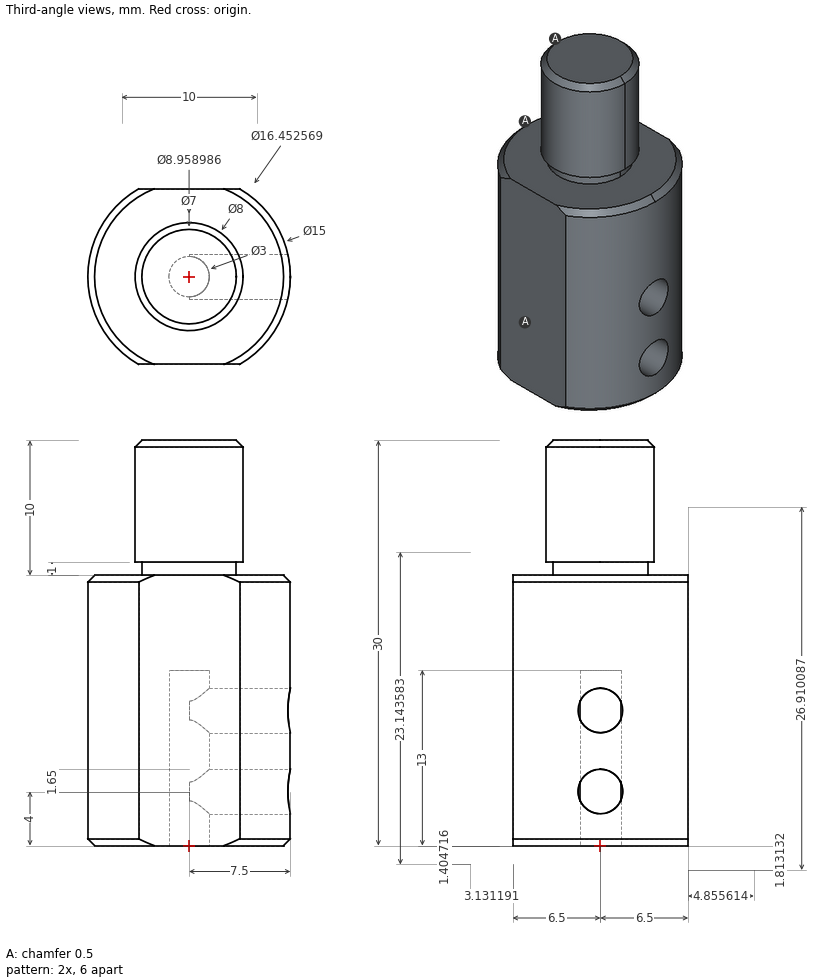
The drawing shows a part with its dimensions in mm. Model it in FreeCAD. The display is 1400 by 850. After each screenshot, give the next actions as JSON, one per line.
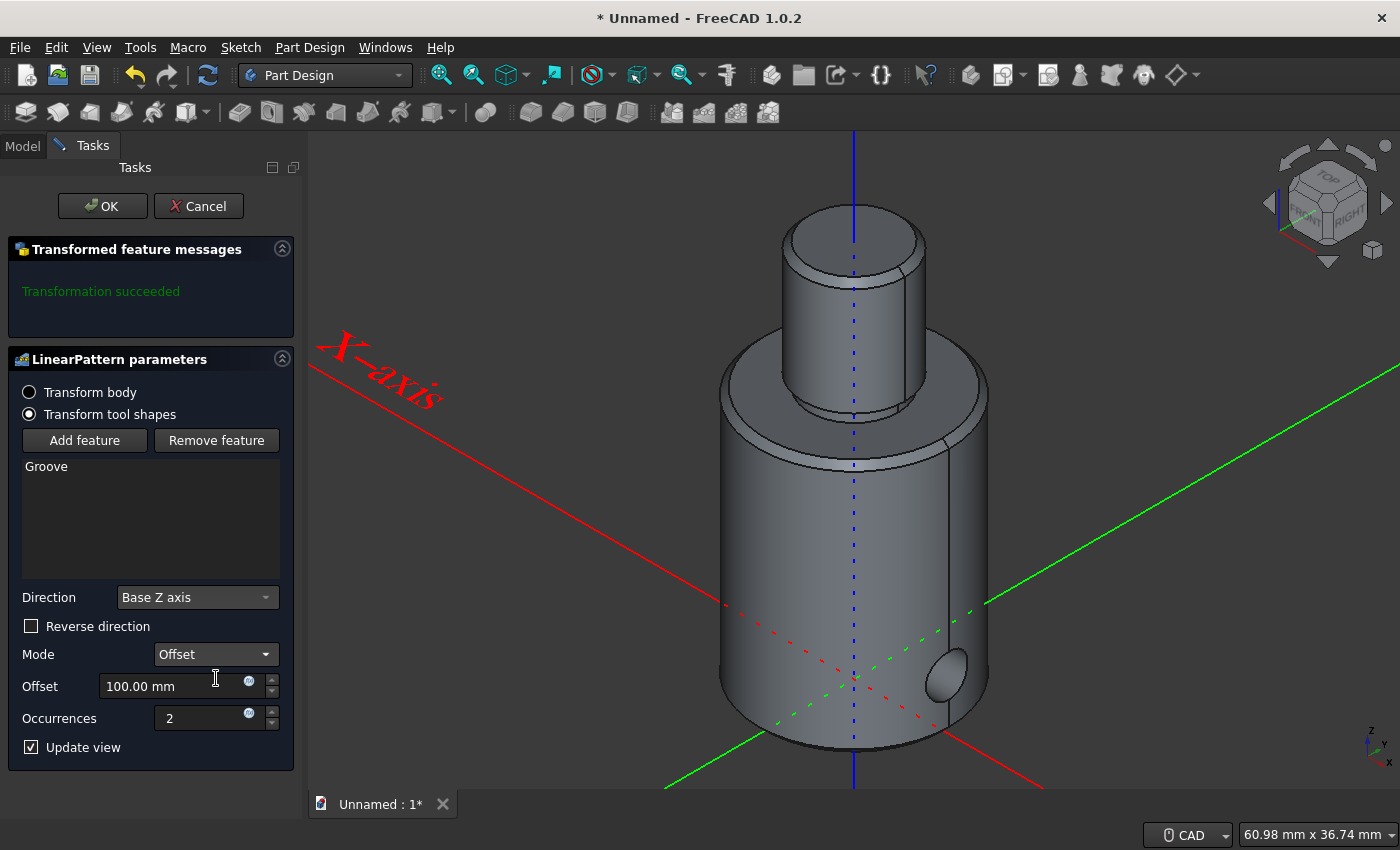
{"action": "triple_click", "coordinate": [182, 686]}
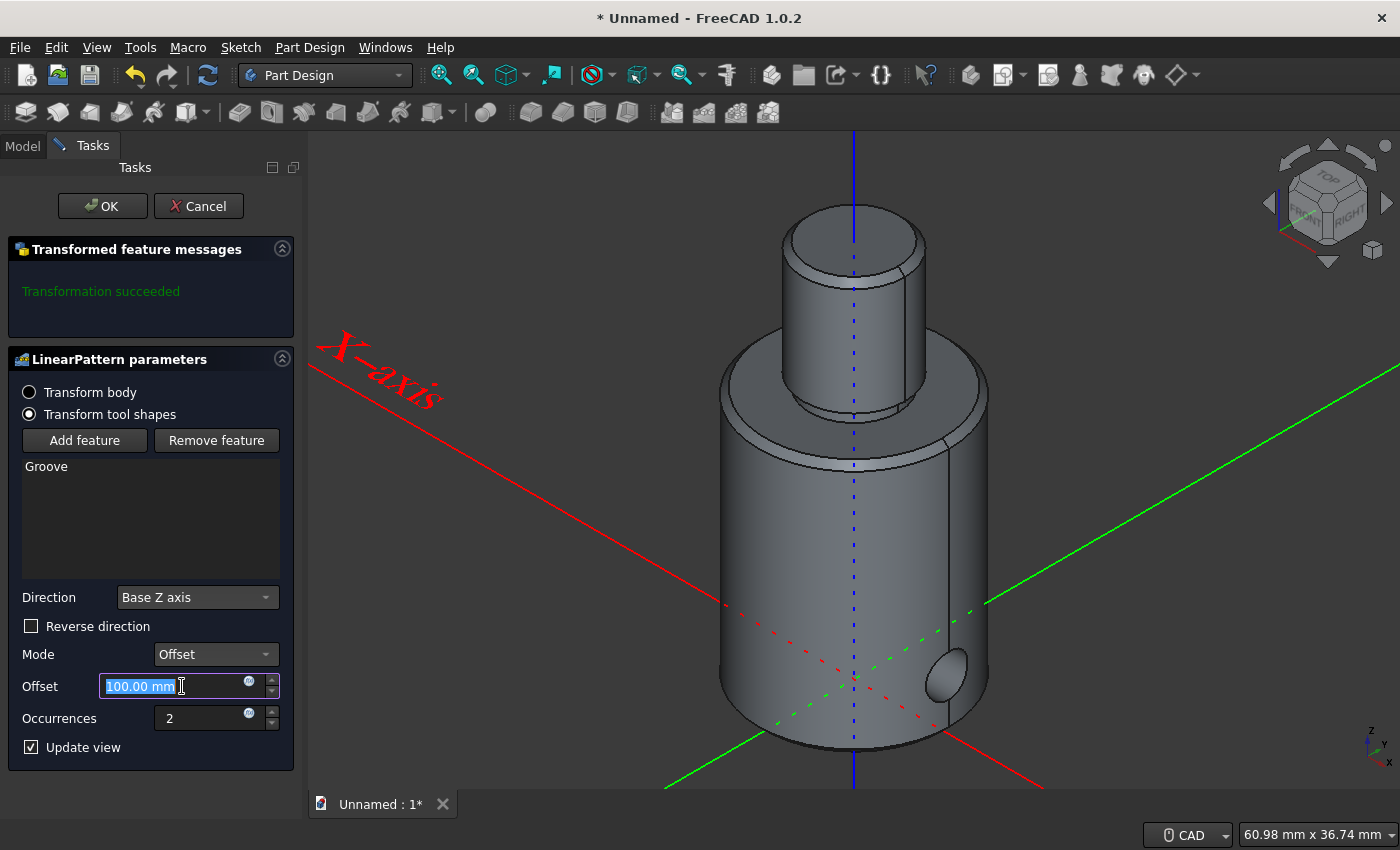
{"action": "type", "text": "6"}
{"action": "key", "text": "Tab"}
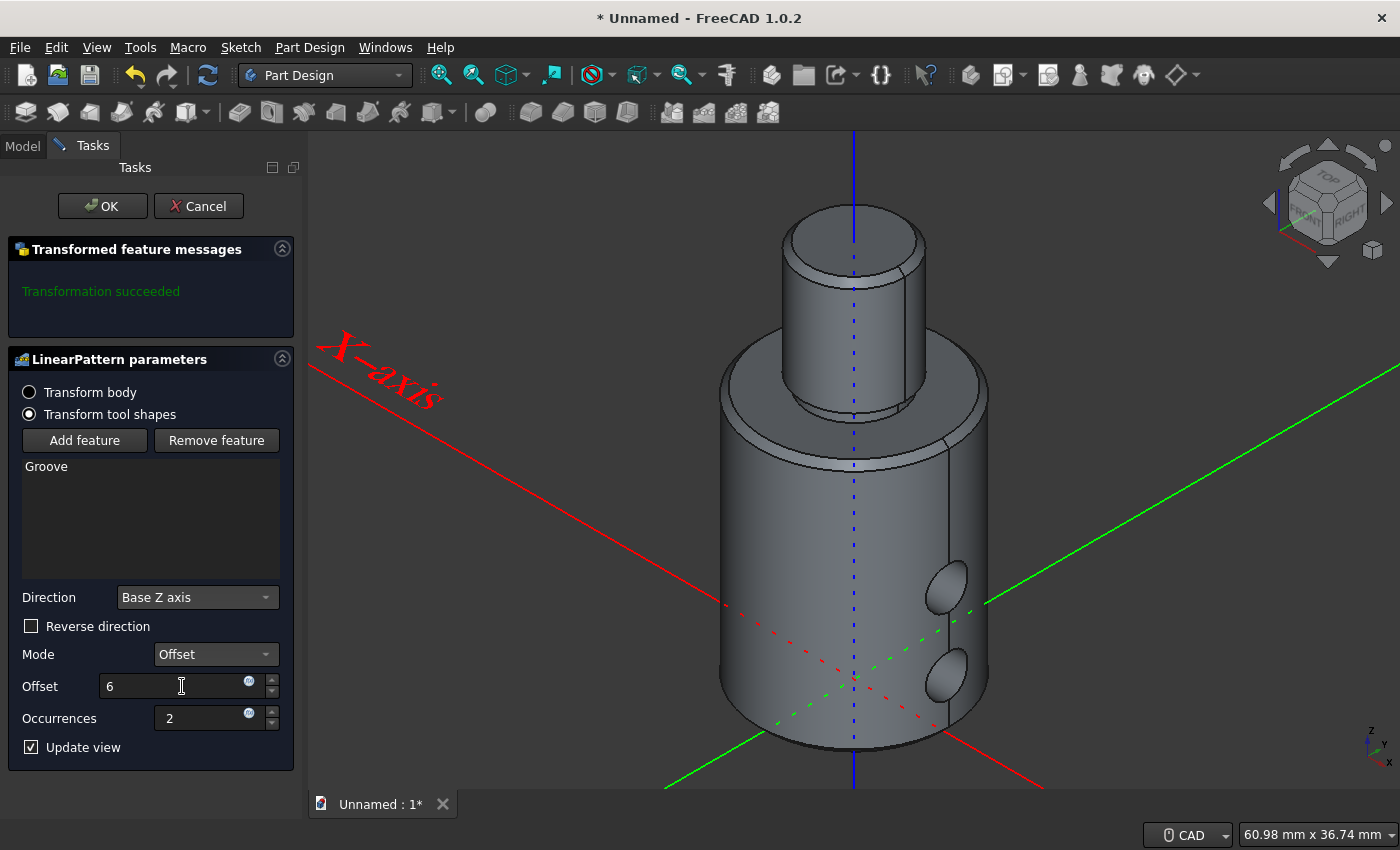
{"action": "triple_click", "coordinate": [209, 718]}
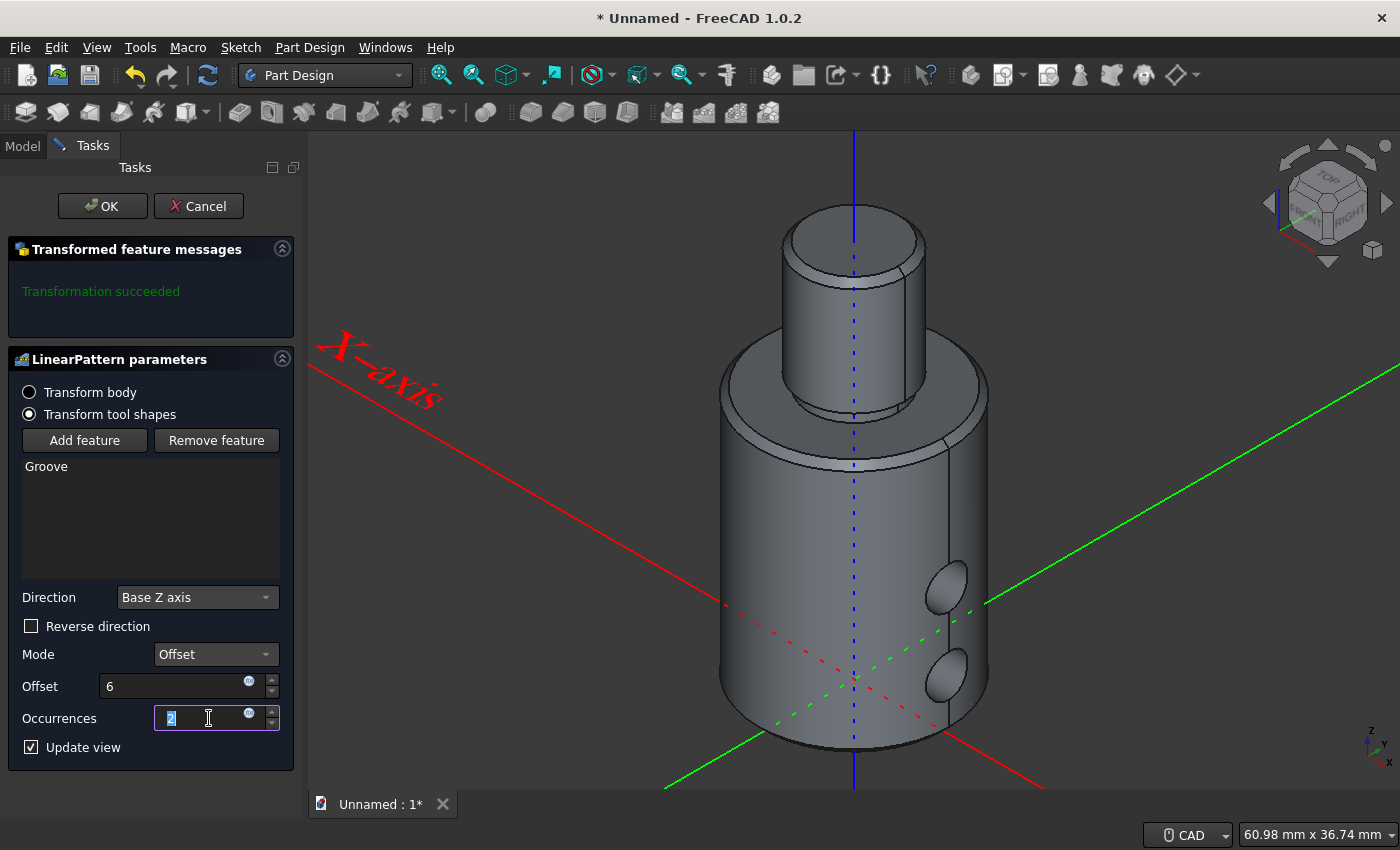
{"action": "type", "text": "2"}
{"action": "key", "text": "Tab"}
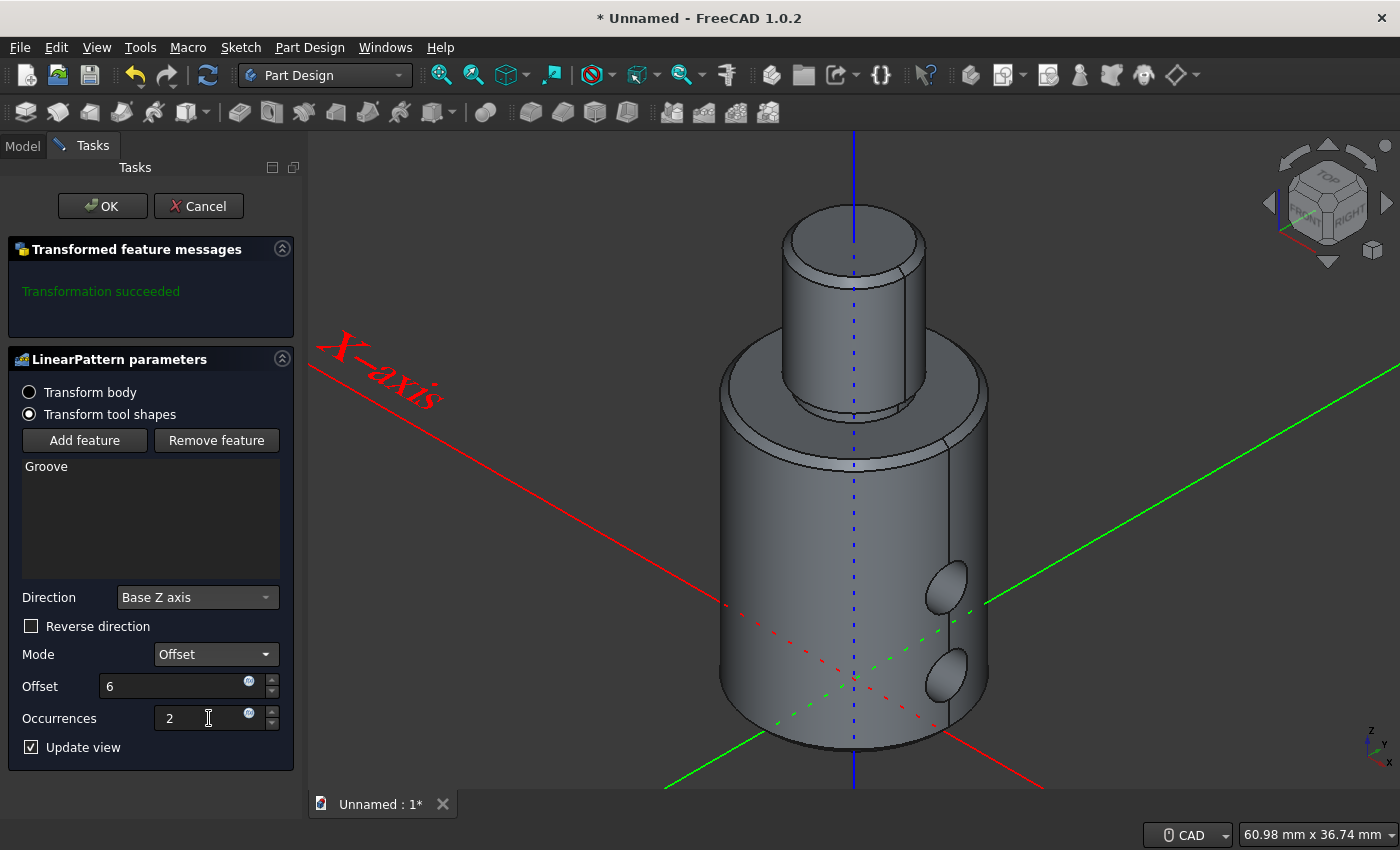
{"action": "left_click", "coordinate": [103, 206]}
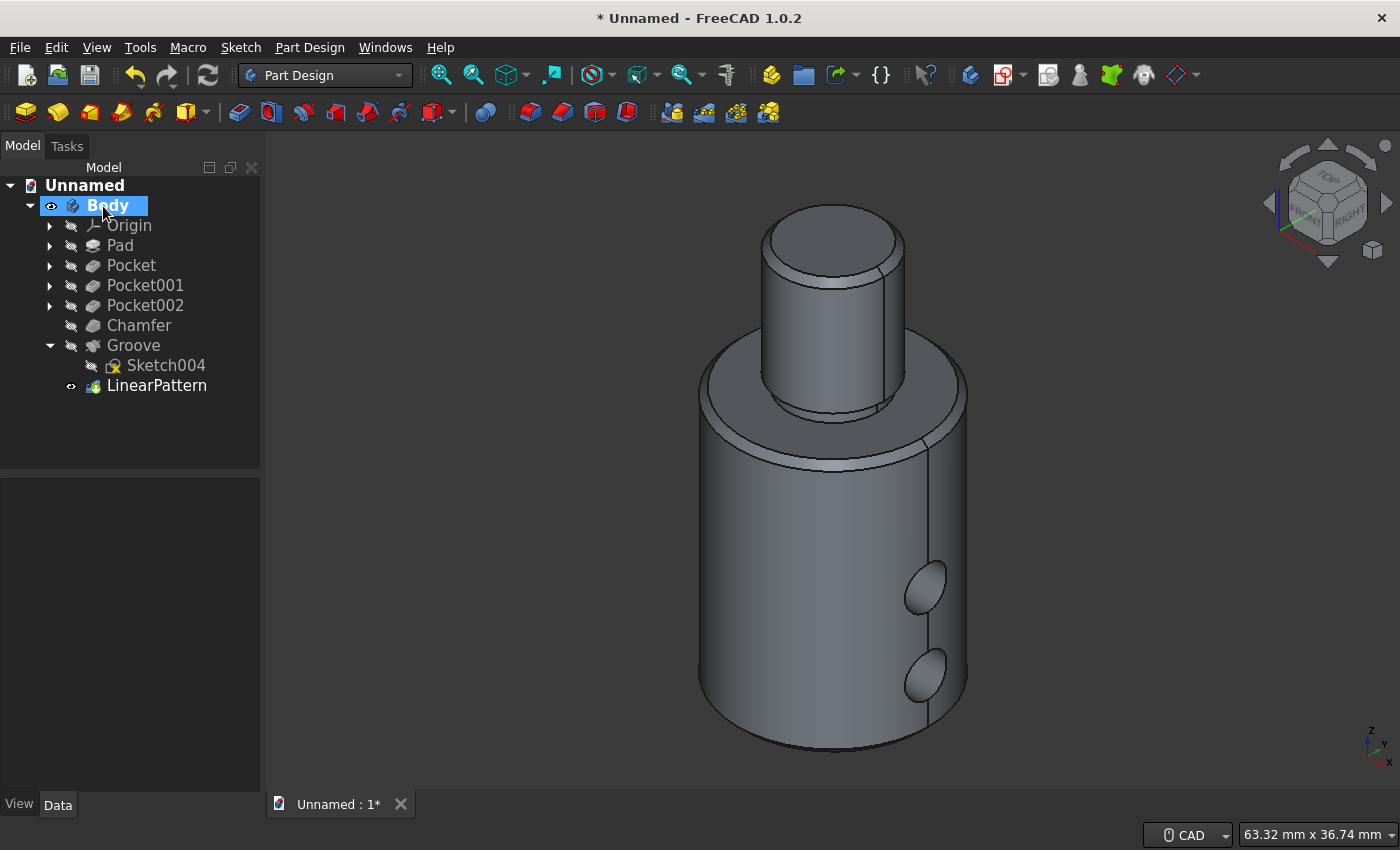
{"action": "left_click", "coordinate": [442, 76]}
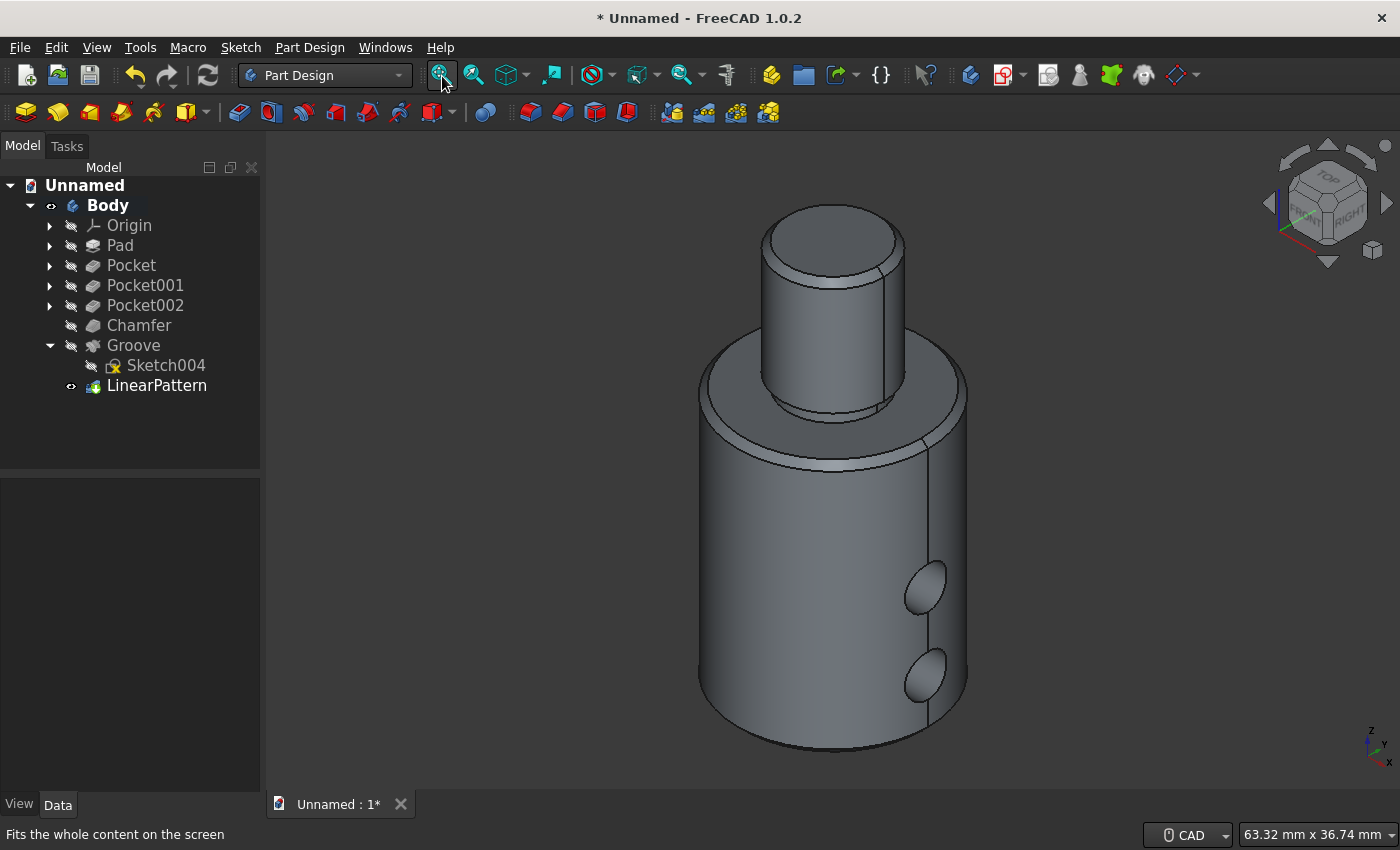
{"action": "left_click", "coordinate": [1004, 76]}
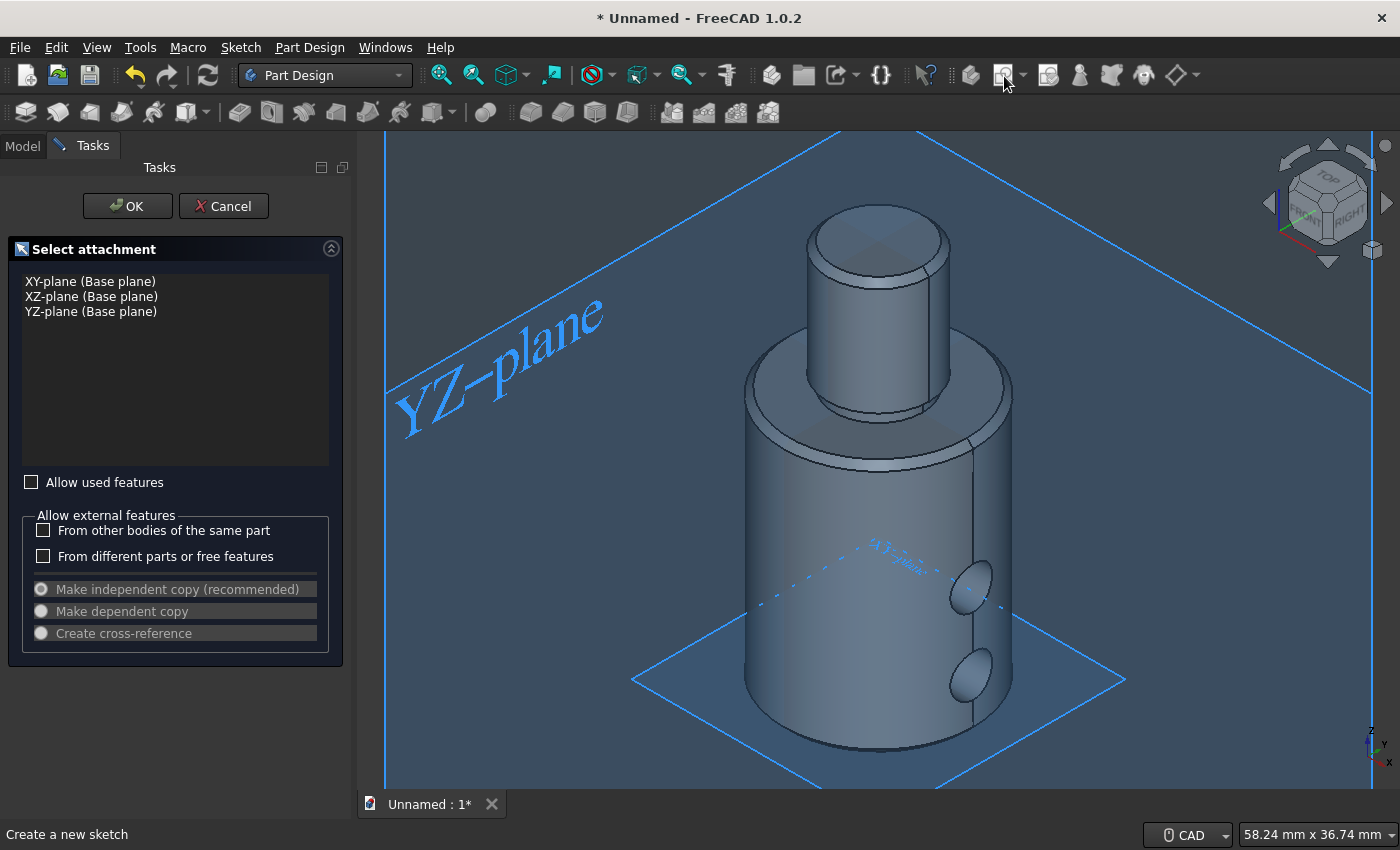
{"action": "left_click", "coordinate": [82, 312]}